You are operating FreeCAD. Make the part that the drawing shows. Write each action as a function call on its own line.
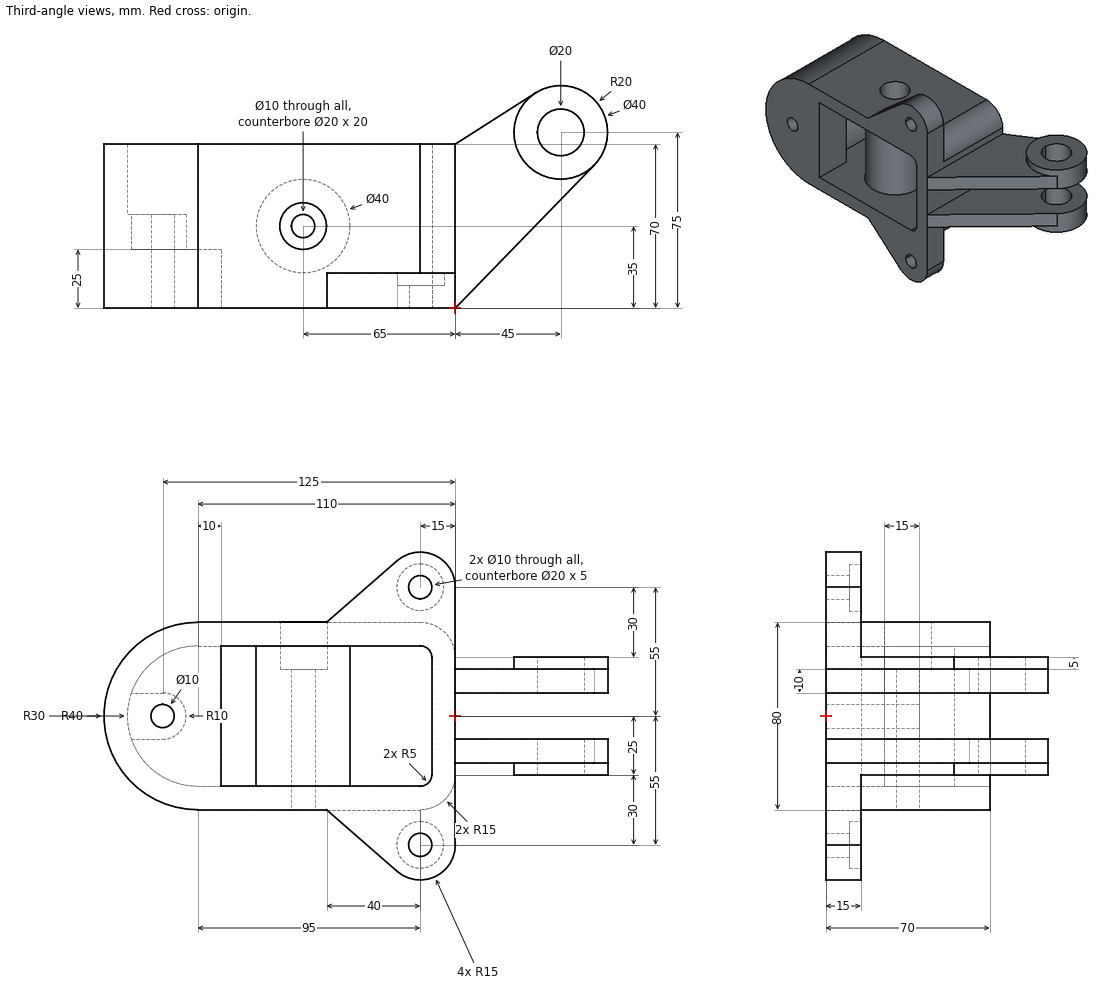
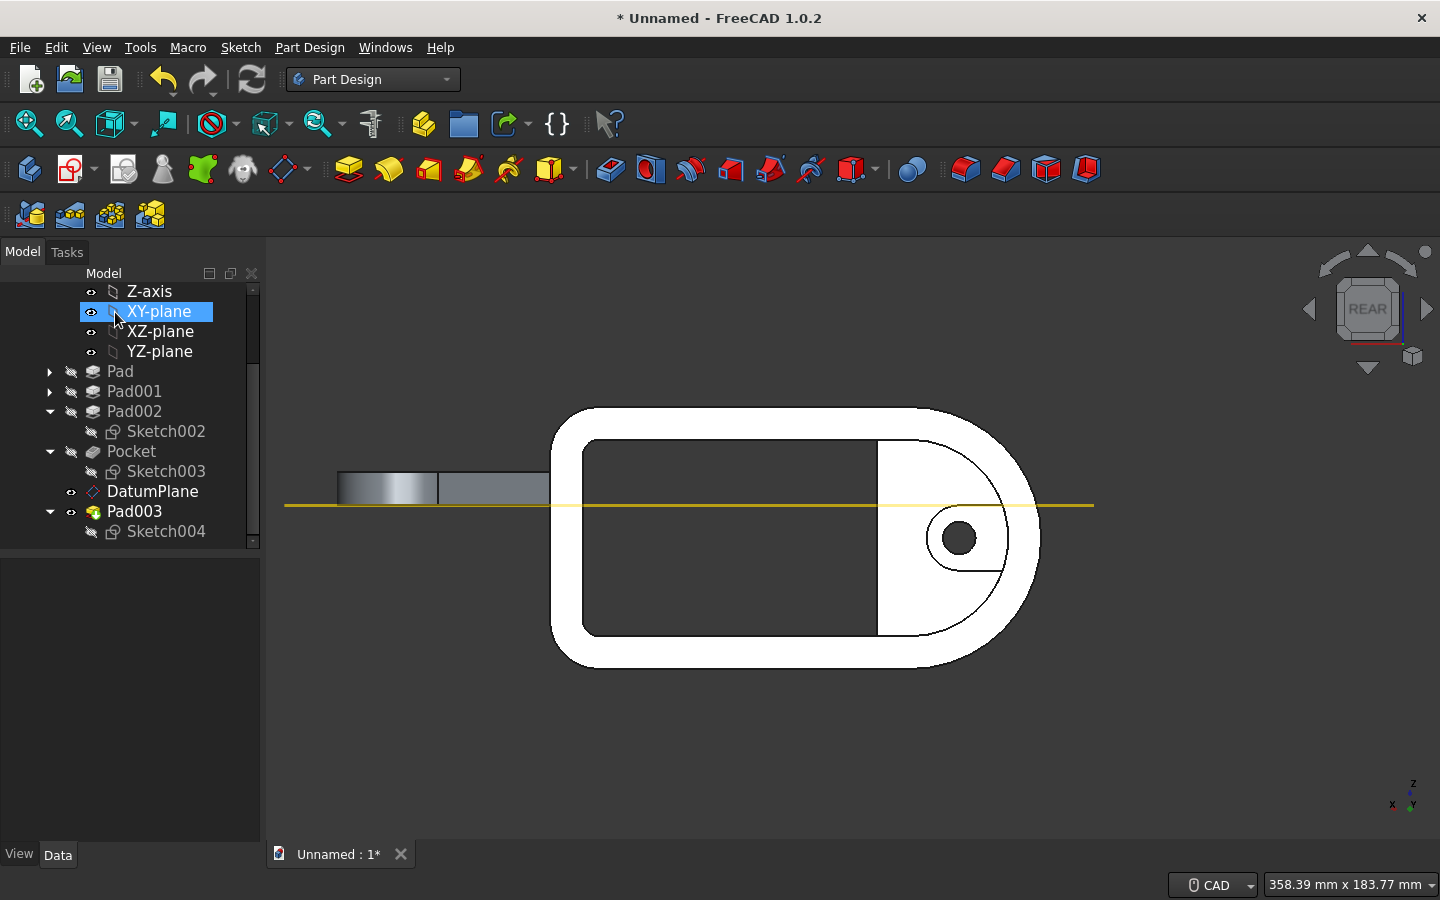
click(116, 492)
key(space)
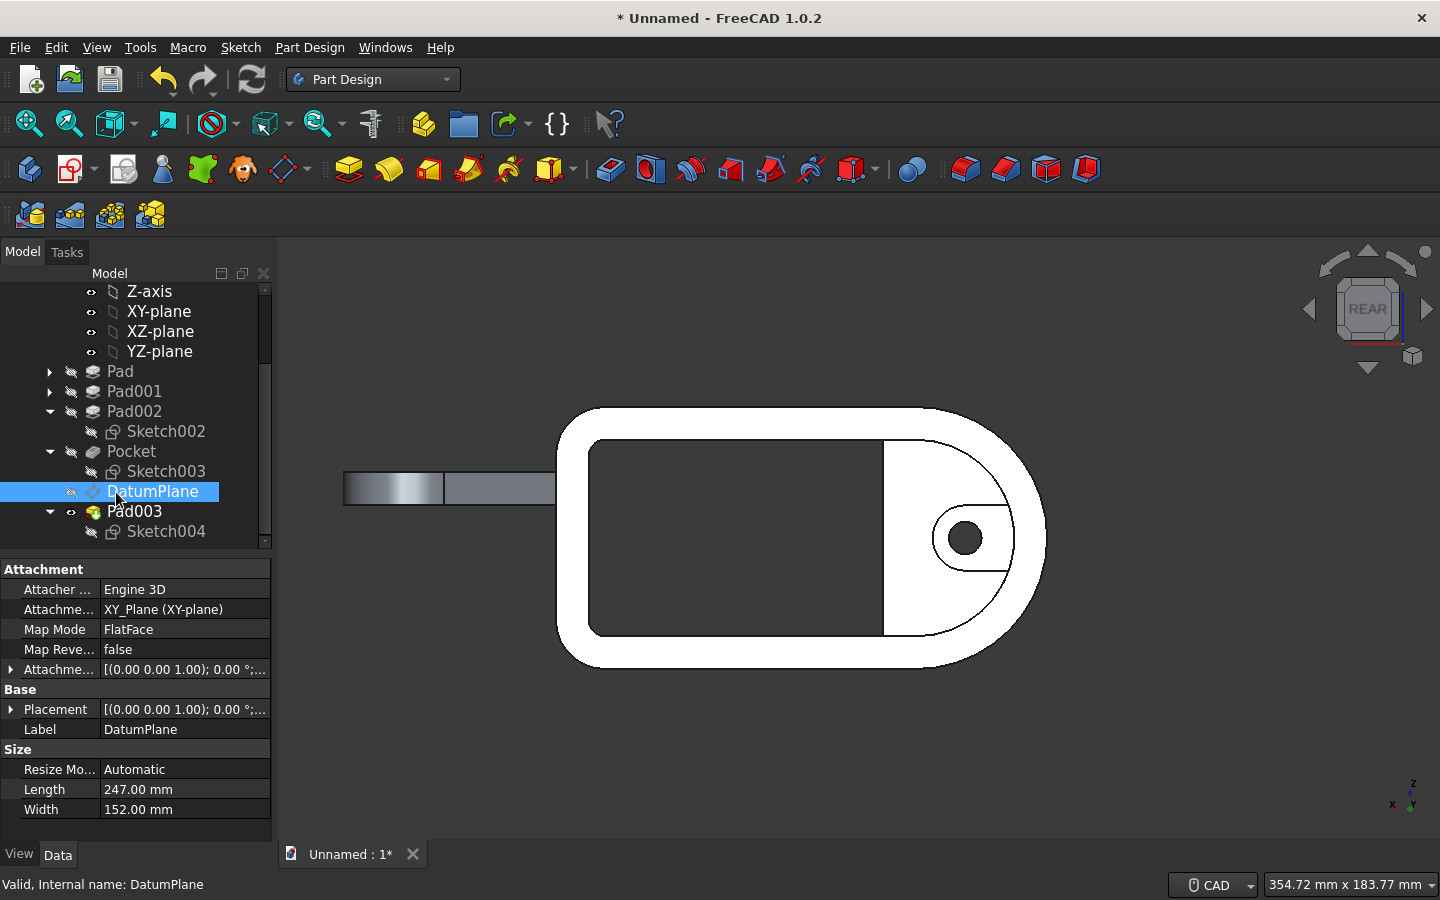
key(0)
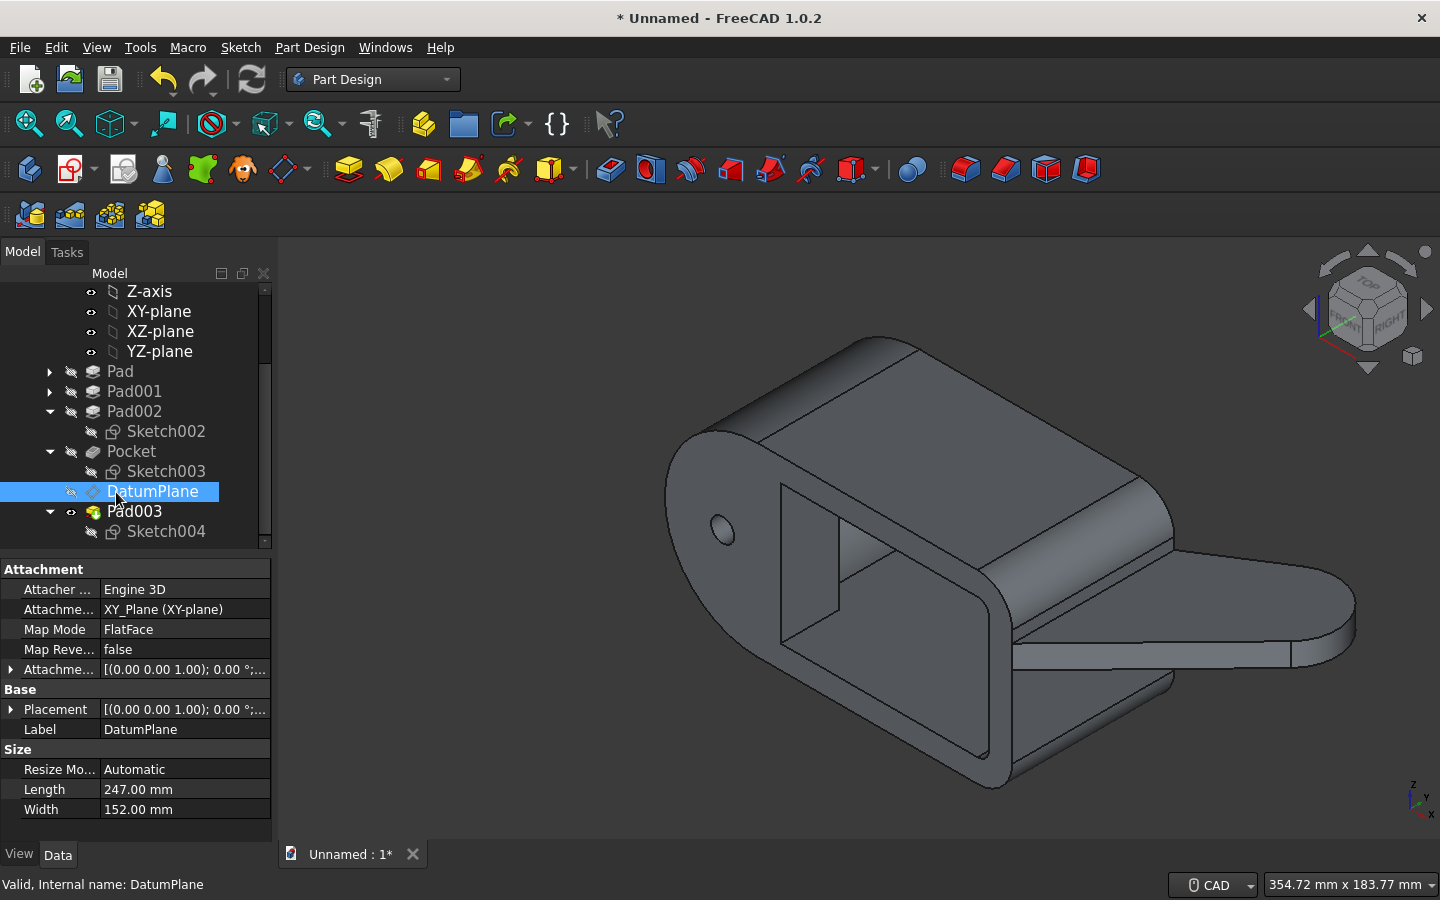
click(30, 124)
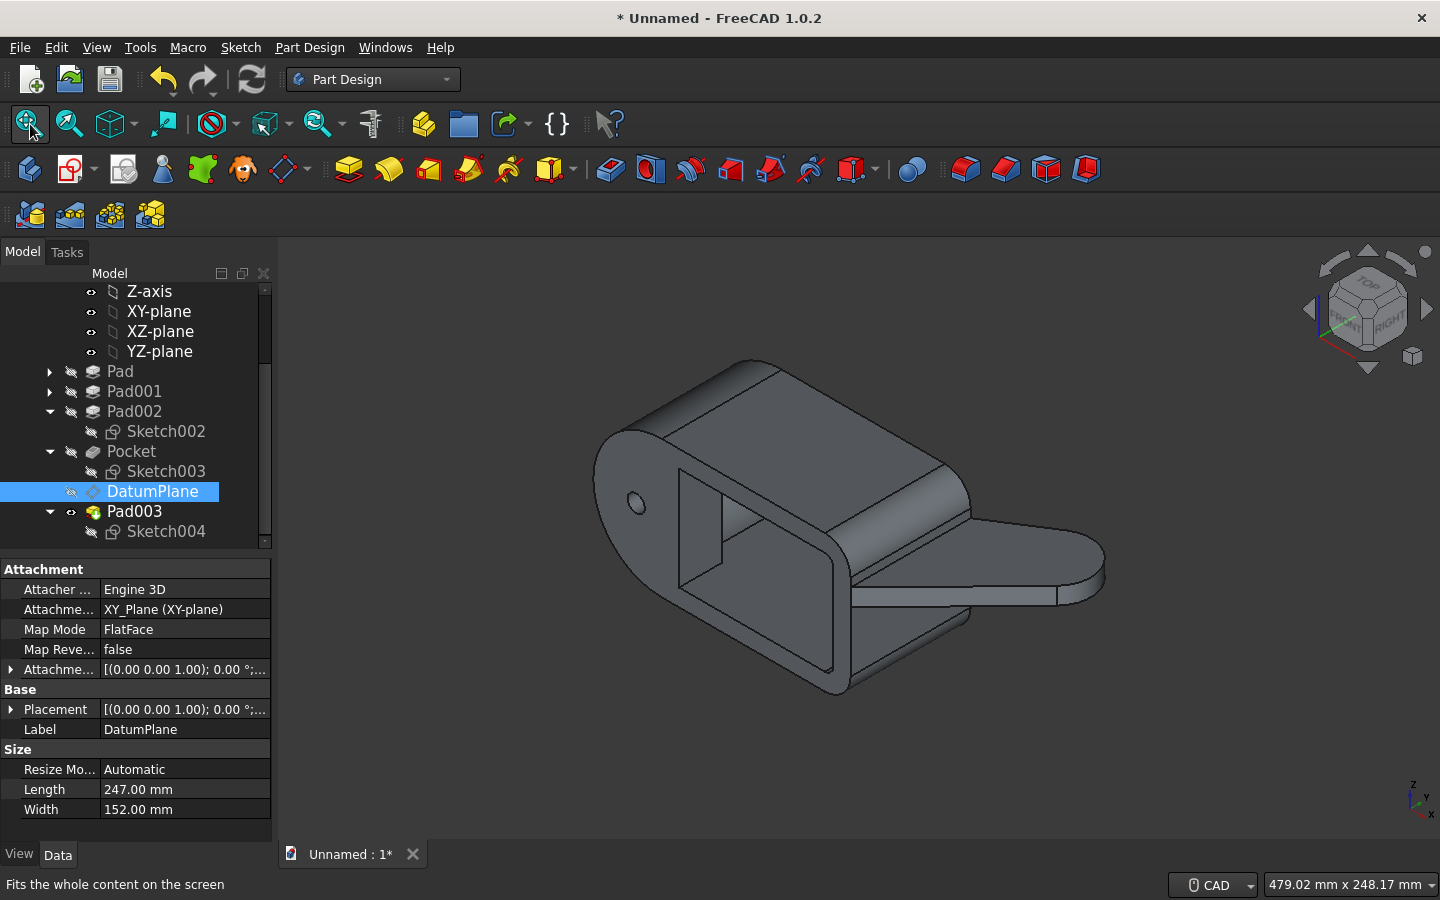
click(995, 549)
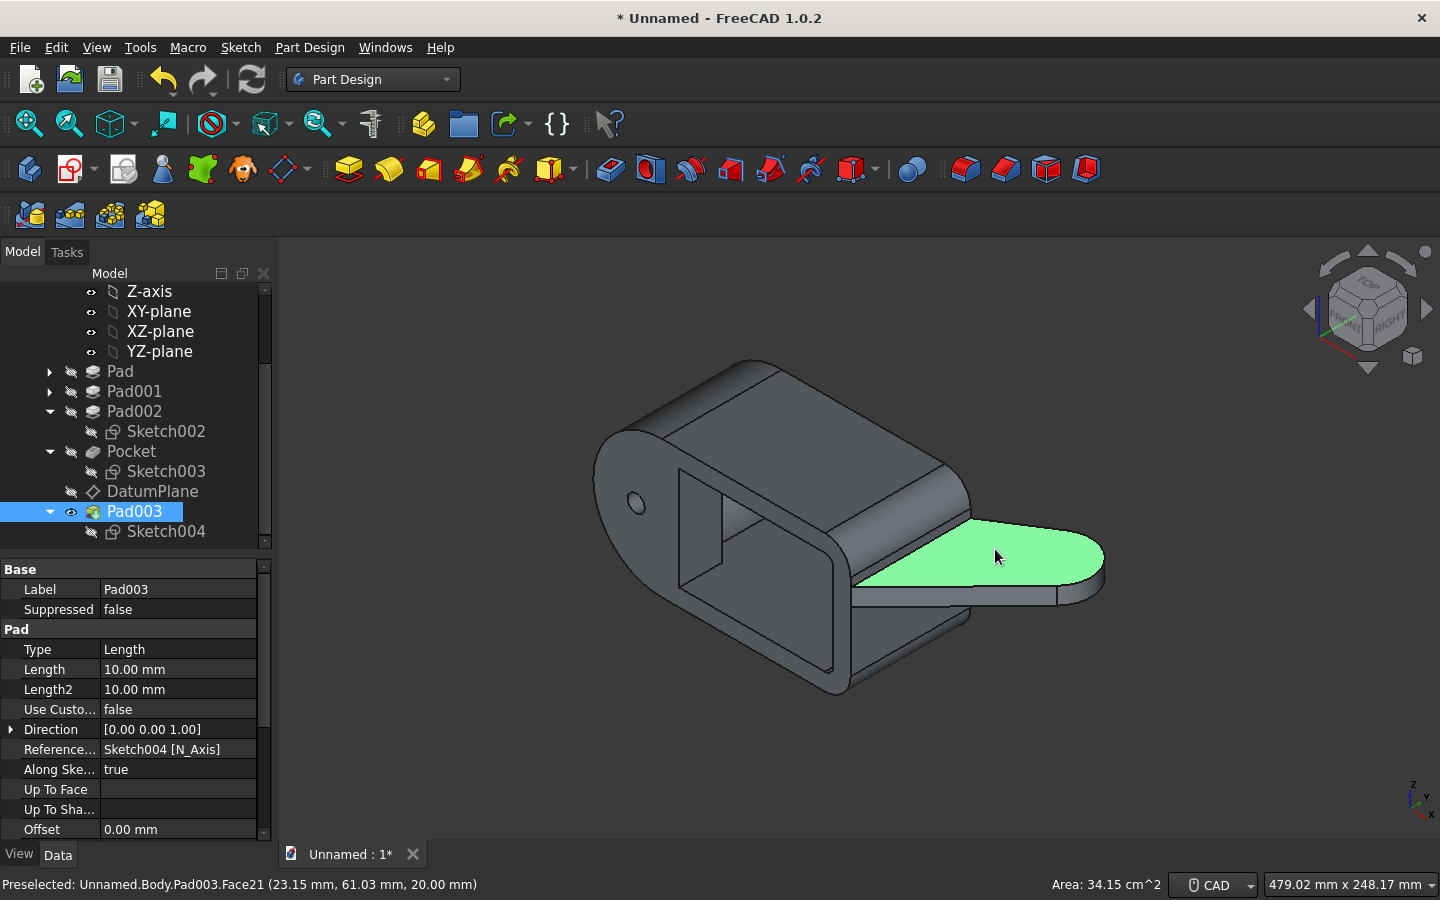
click(70, 170)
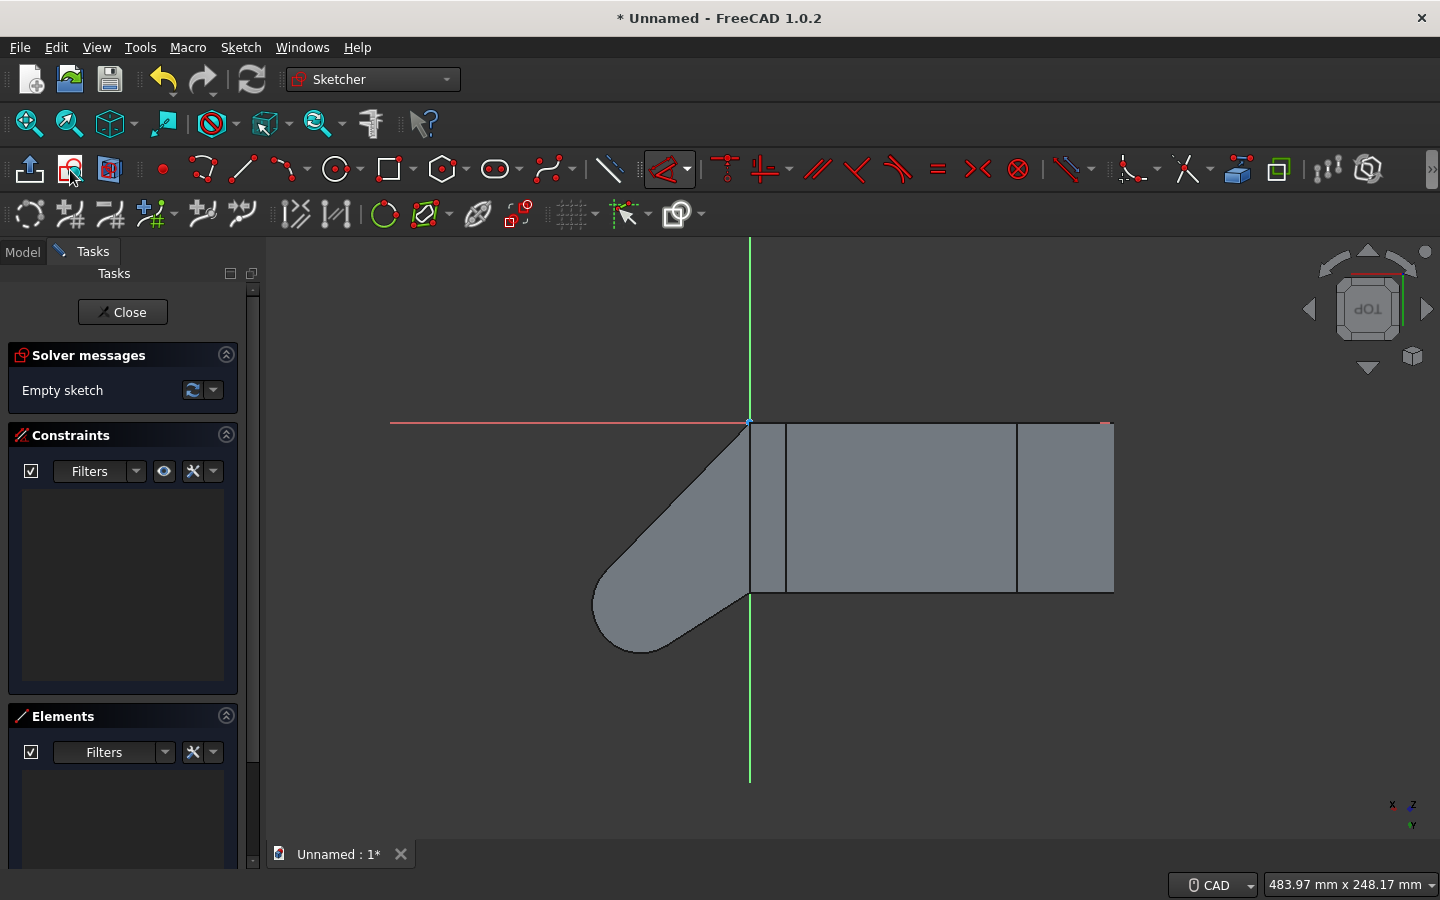
scroll(533, 538, up, 3)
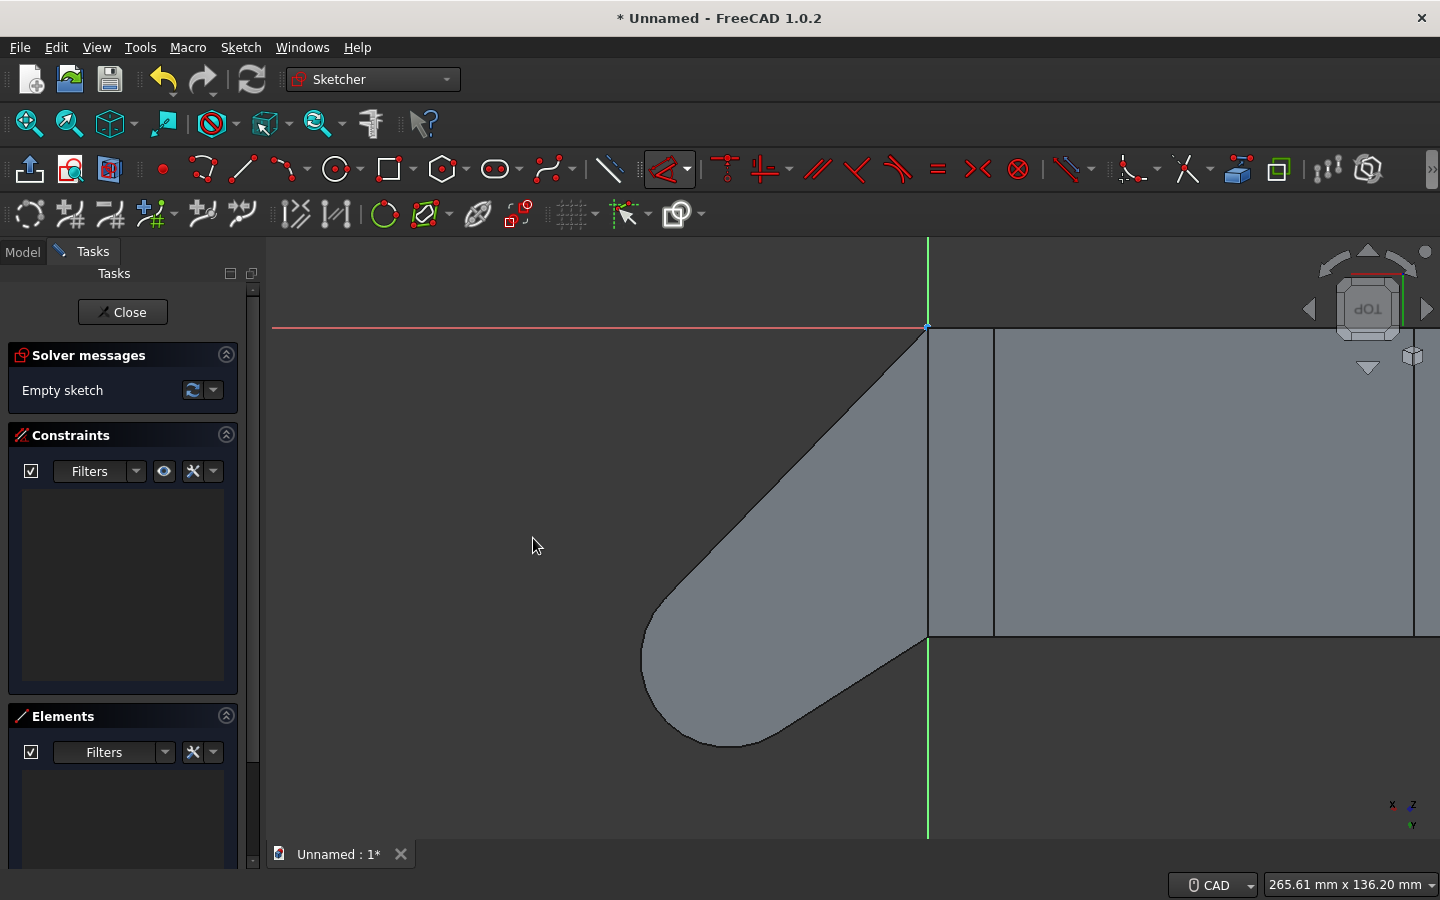
key(g)
key(c)